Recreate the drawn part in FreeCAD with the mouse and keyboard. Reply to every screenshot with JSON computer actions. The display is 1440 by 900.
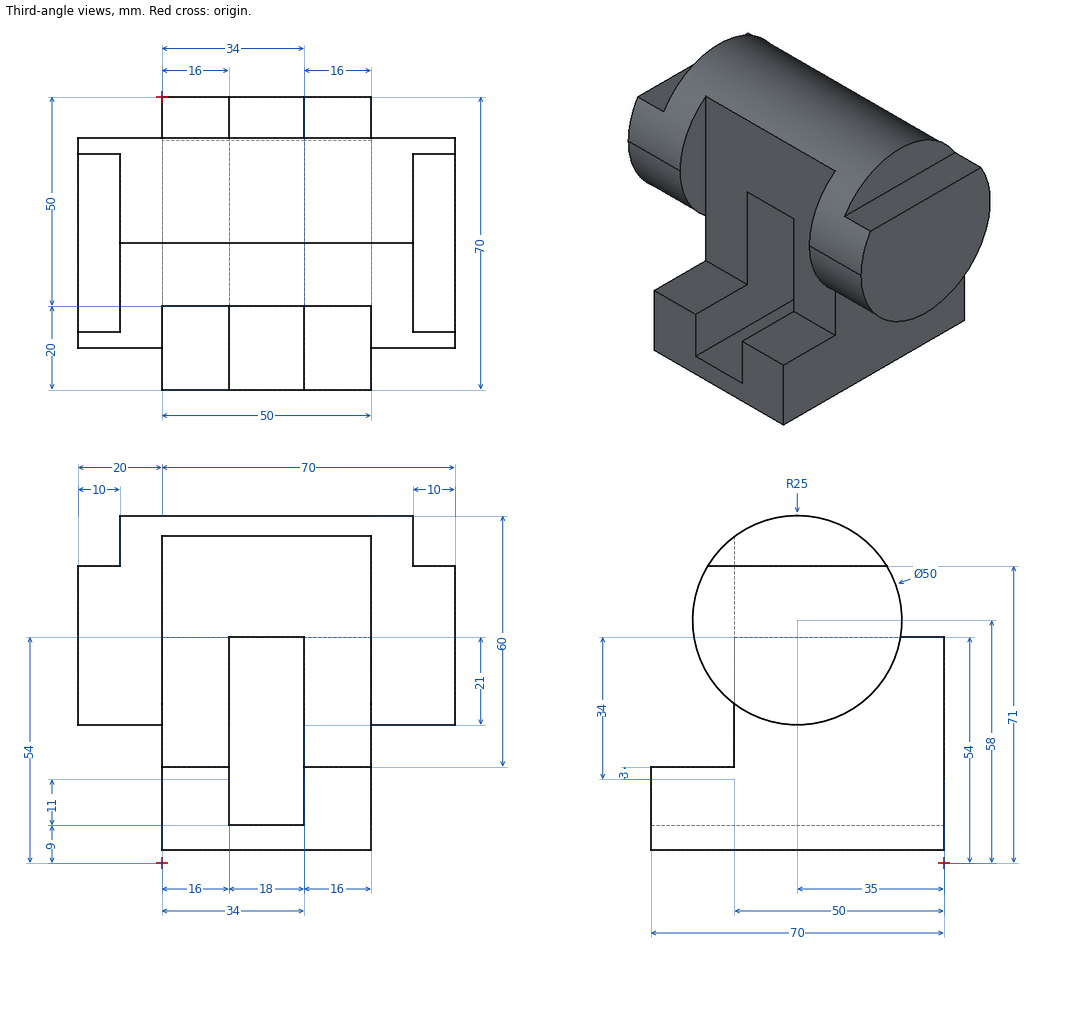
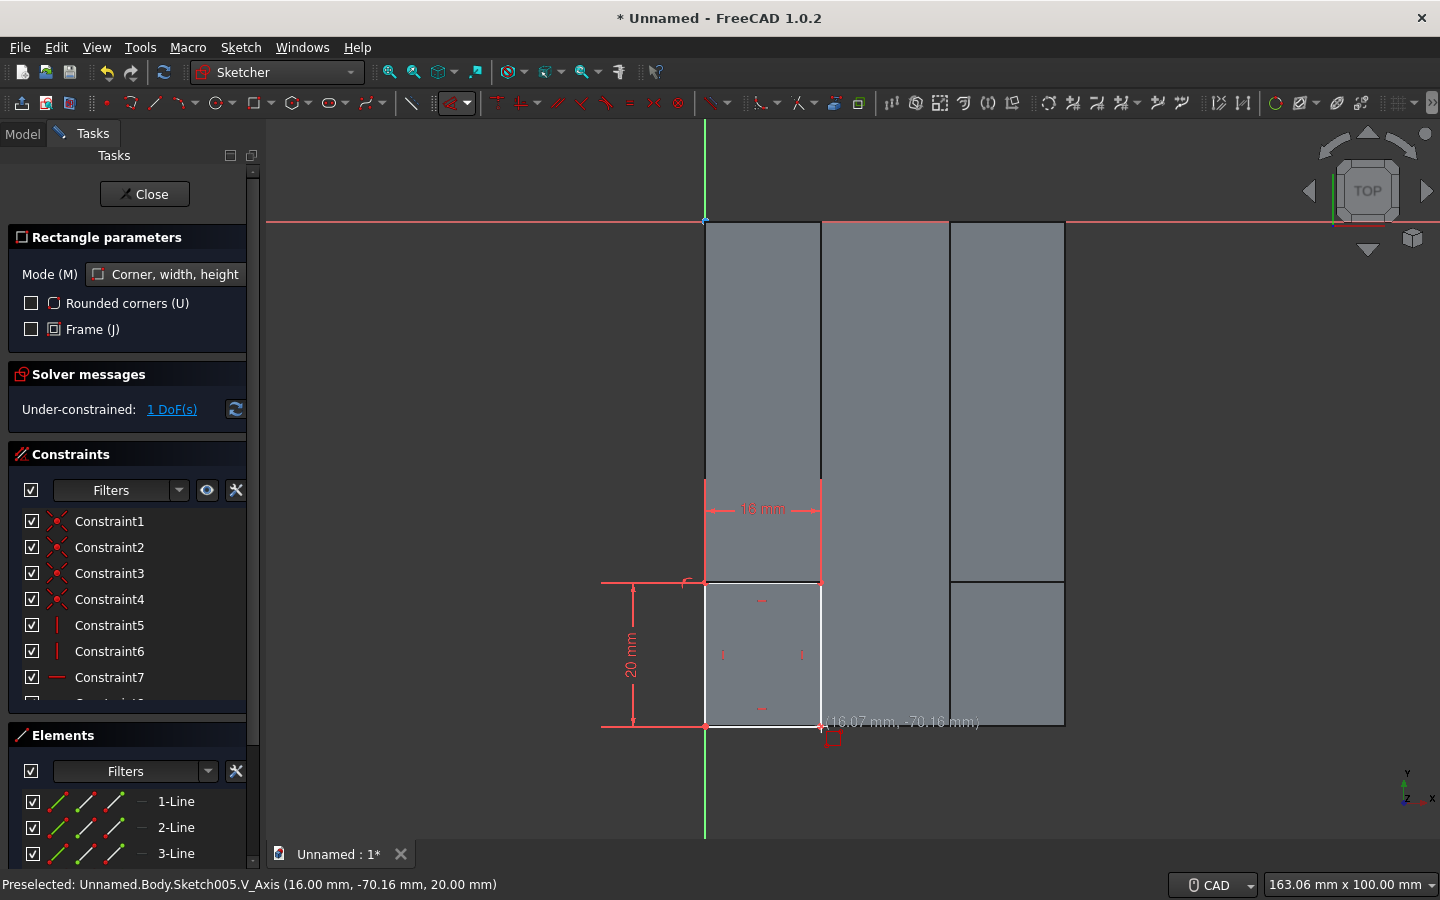
{"action": "left_click", "coordinate": [950, 582]}
{"action": "mouse_move", "coordinate": [1065, 726]}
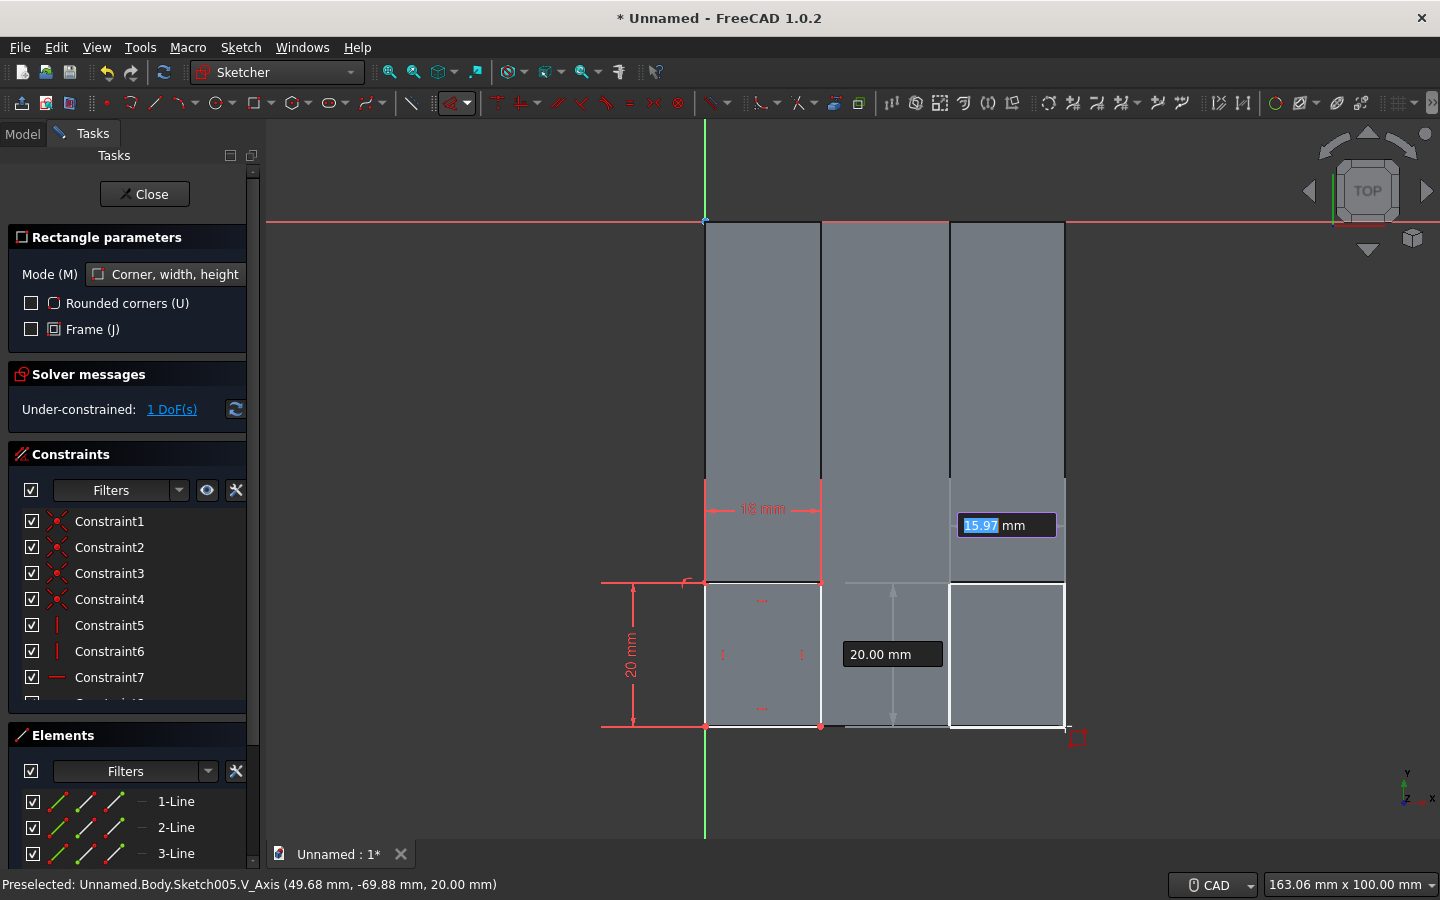
{"action": "type", "text": "16"}
{"action": "key", "text": "Tab"}
{"action": "type", "text": "20"}
{"action": "key", "text": "Return"}
{"action": "key", "text": "Escape"}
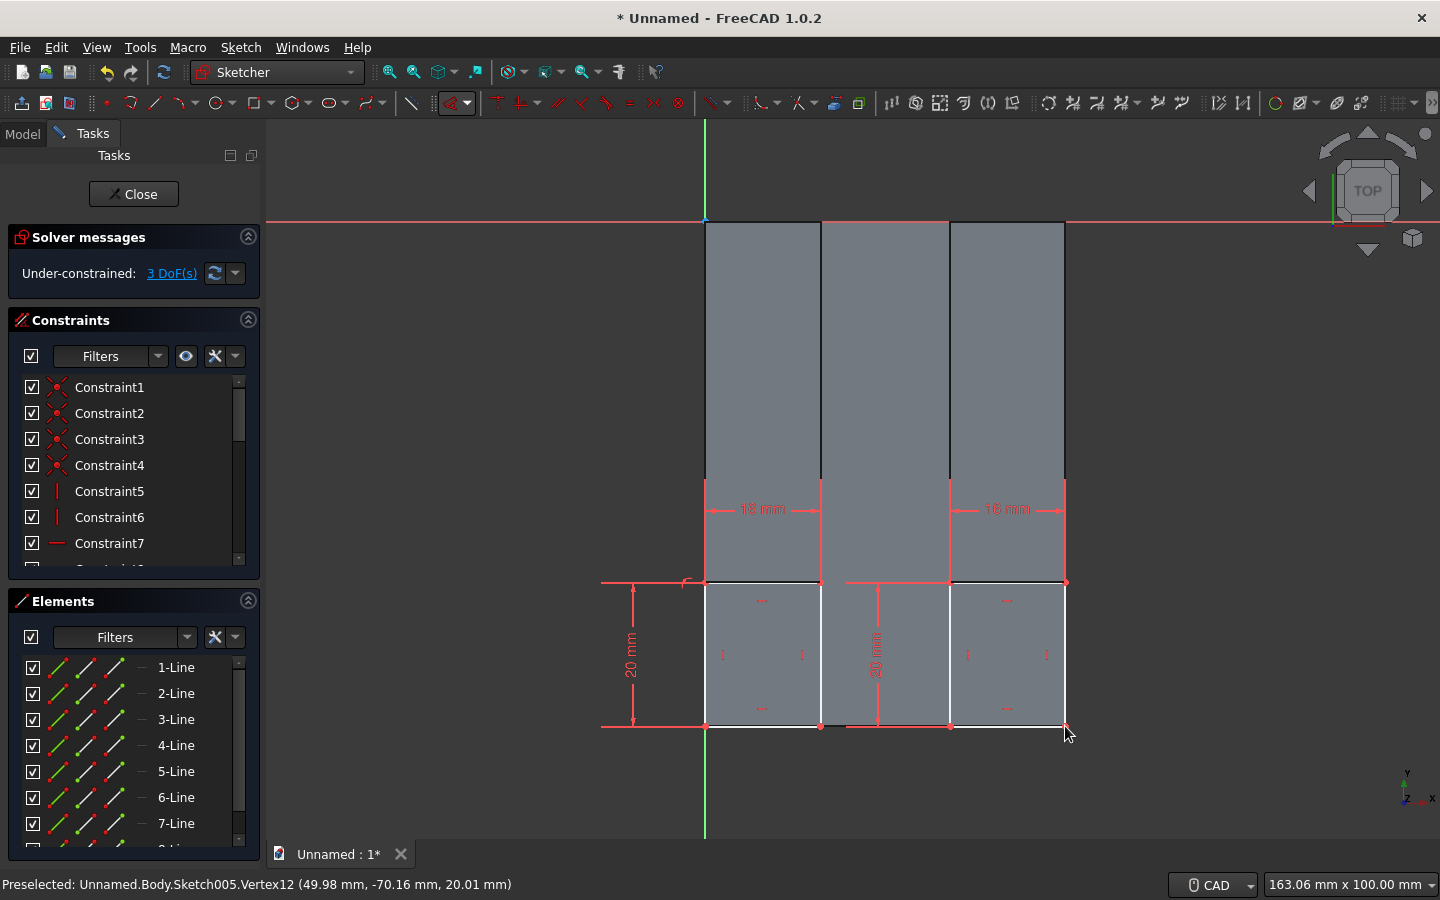
{"action": "left_click", "coordinate": [705, 583]}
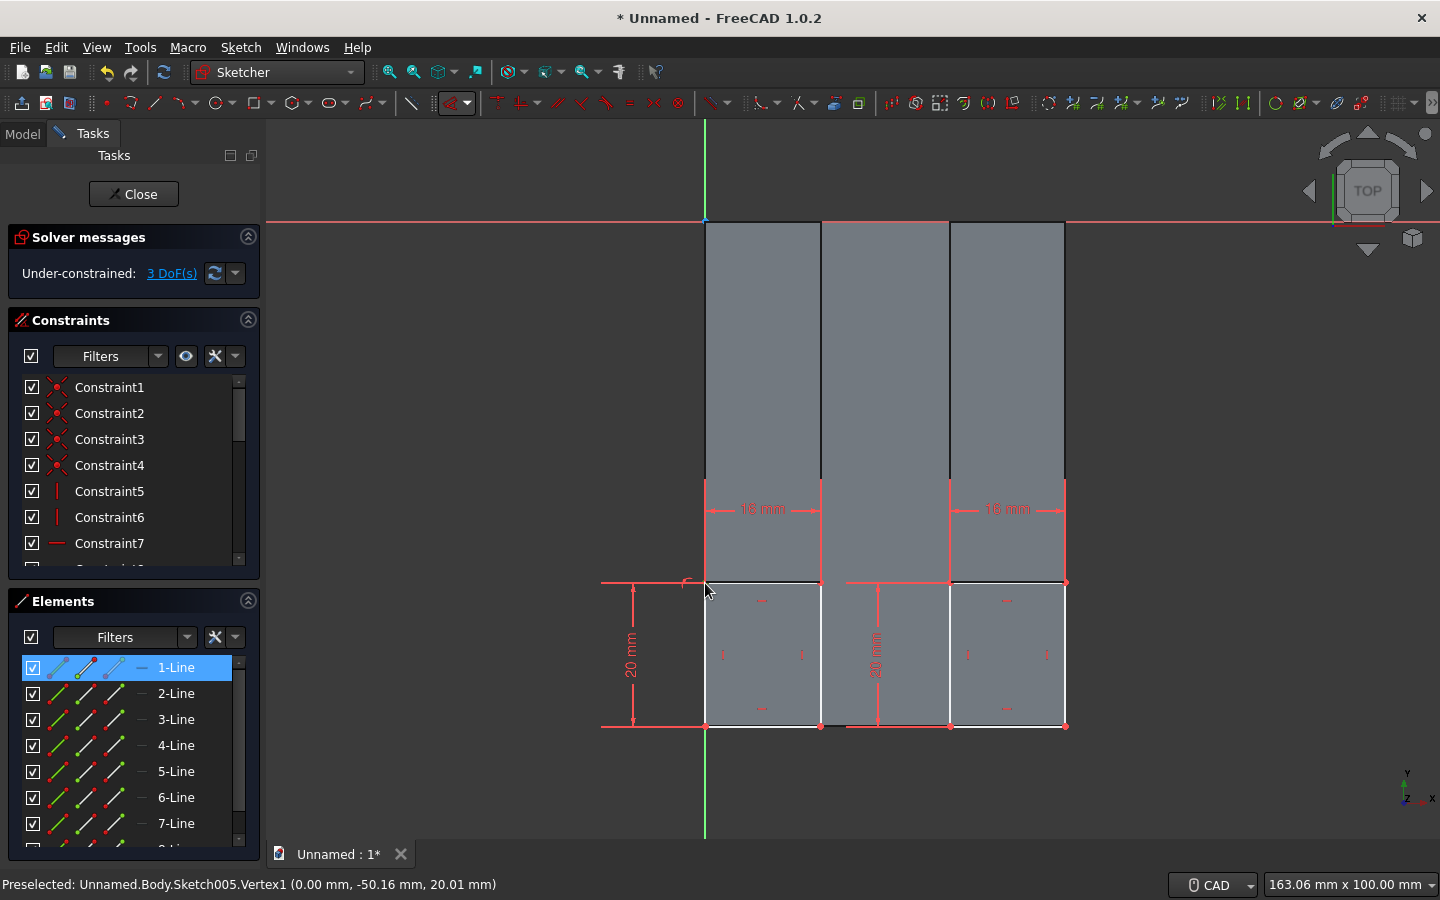
{"action": "key", "text": "i"}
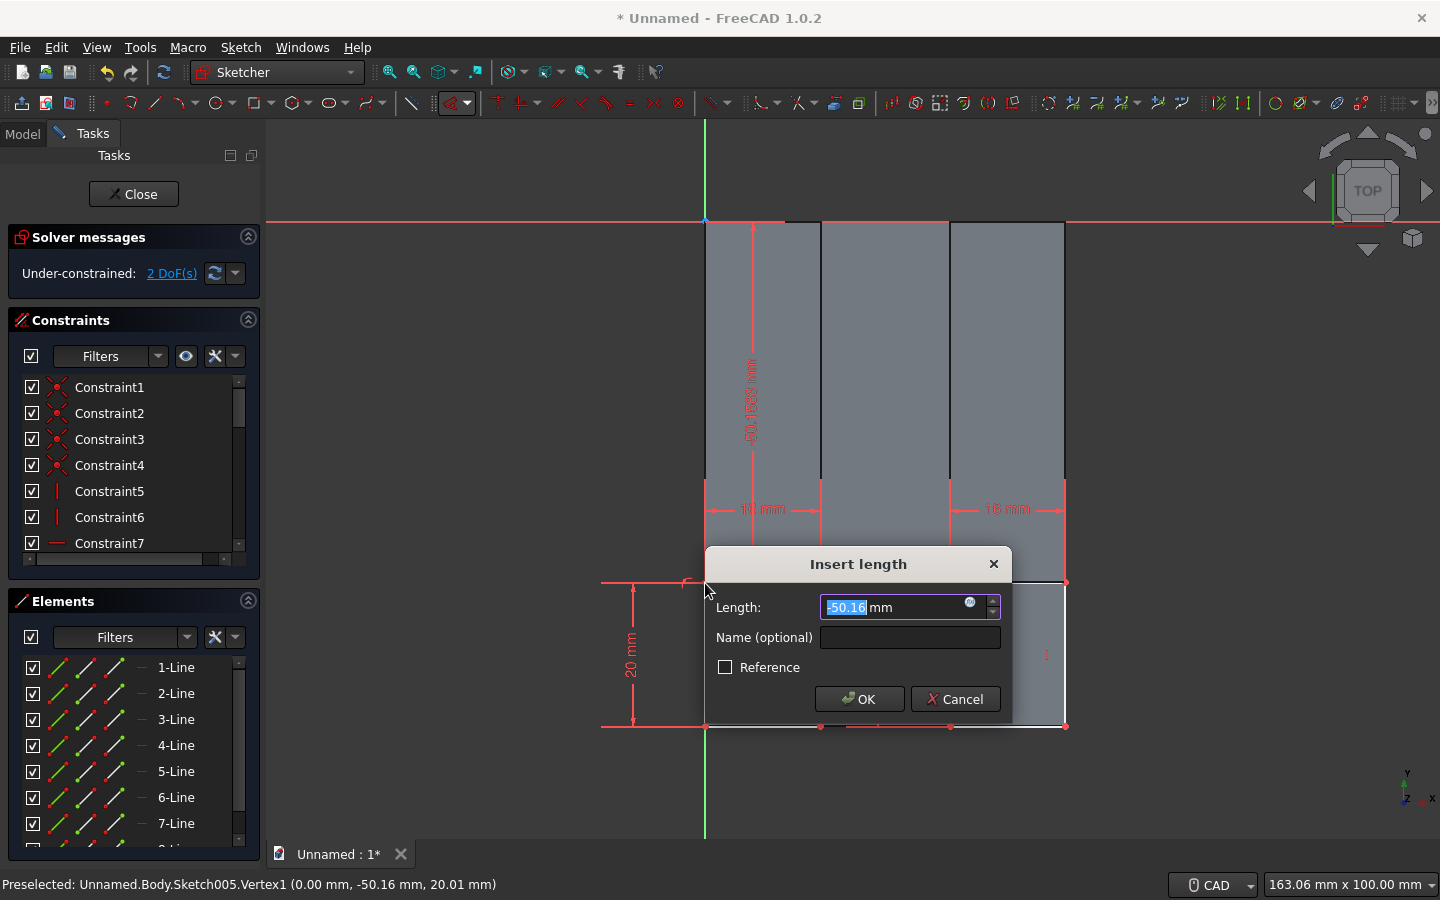
{"action": "type", "text": "-50"}
{"action": "key", "text": "Return"}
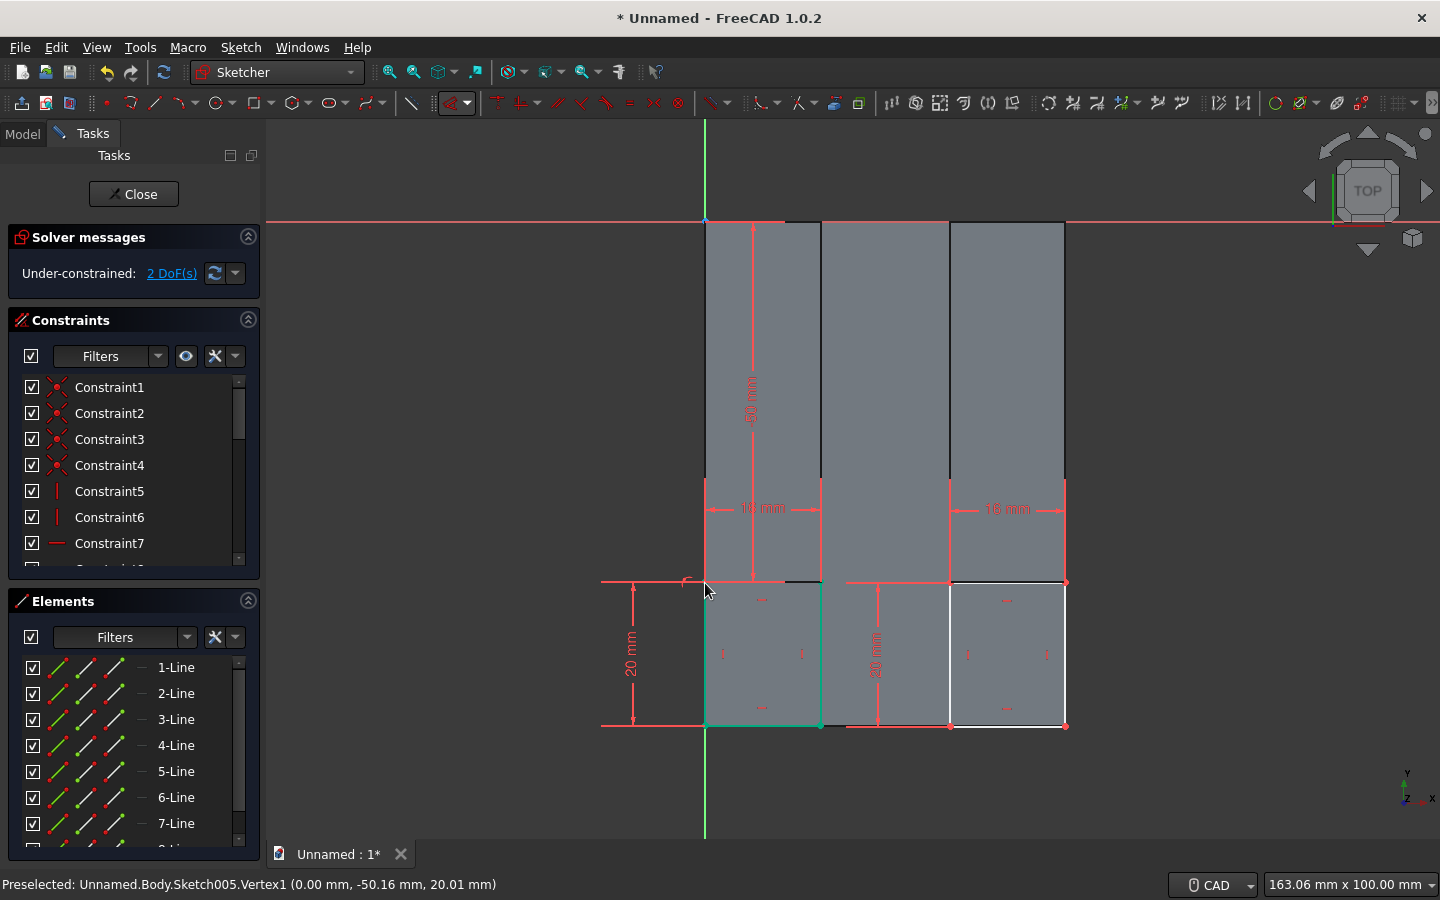
{"action": "left_click", "coordinate": [950, 583]}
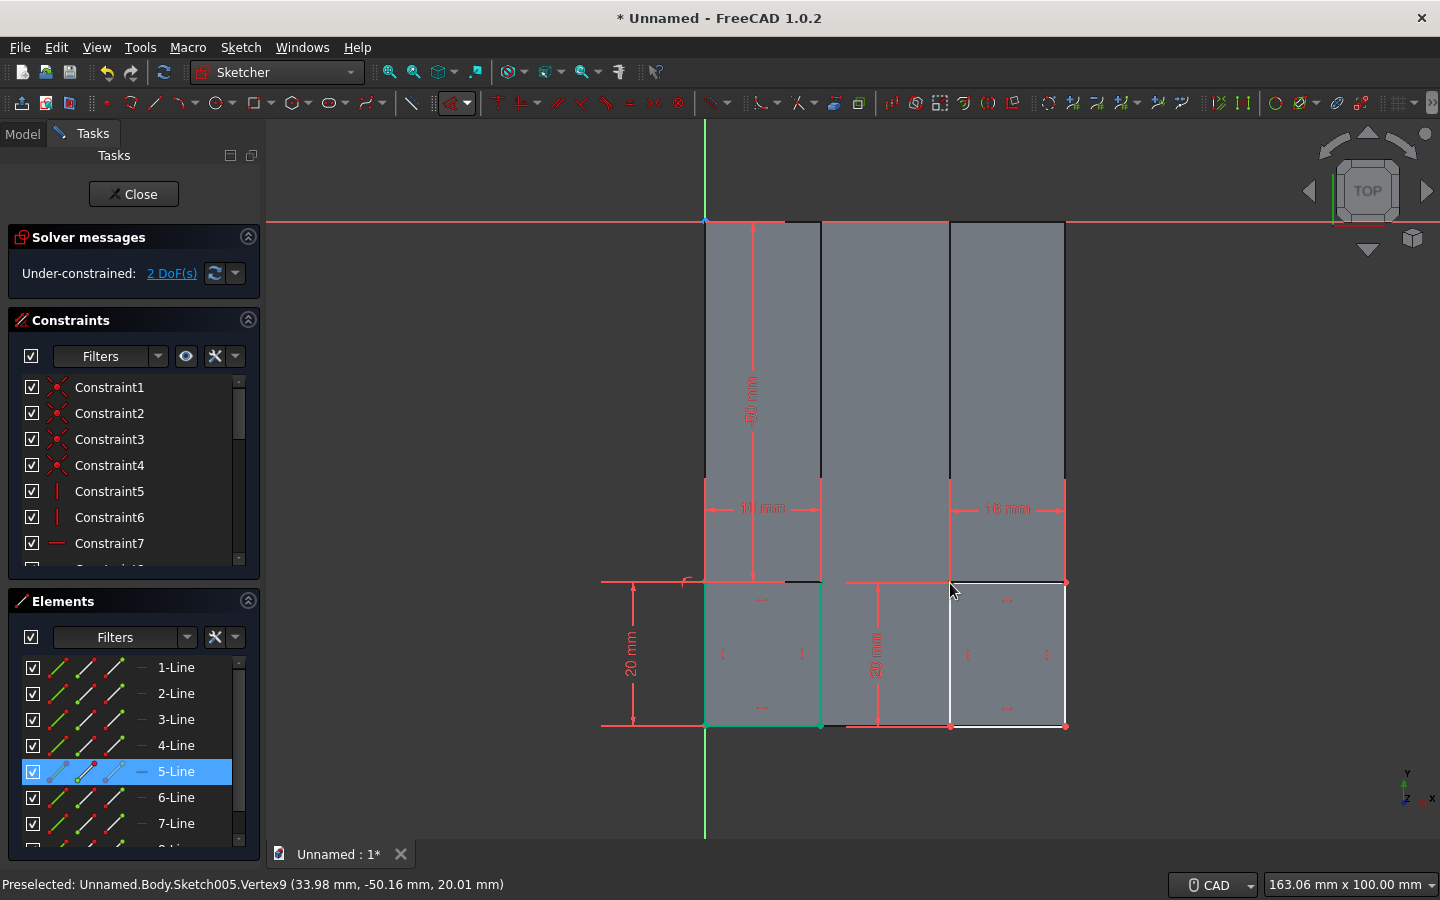
{"action": "key", "text": "l"}